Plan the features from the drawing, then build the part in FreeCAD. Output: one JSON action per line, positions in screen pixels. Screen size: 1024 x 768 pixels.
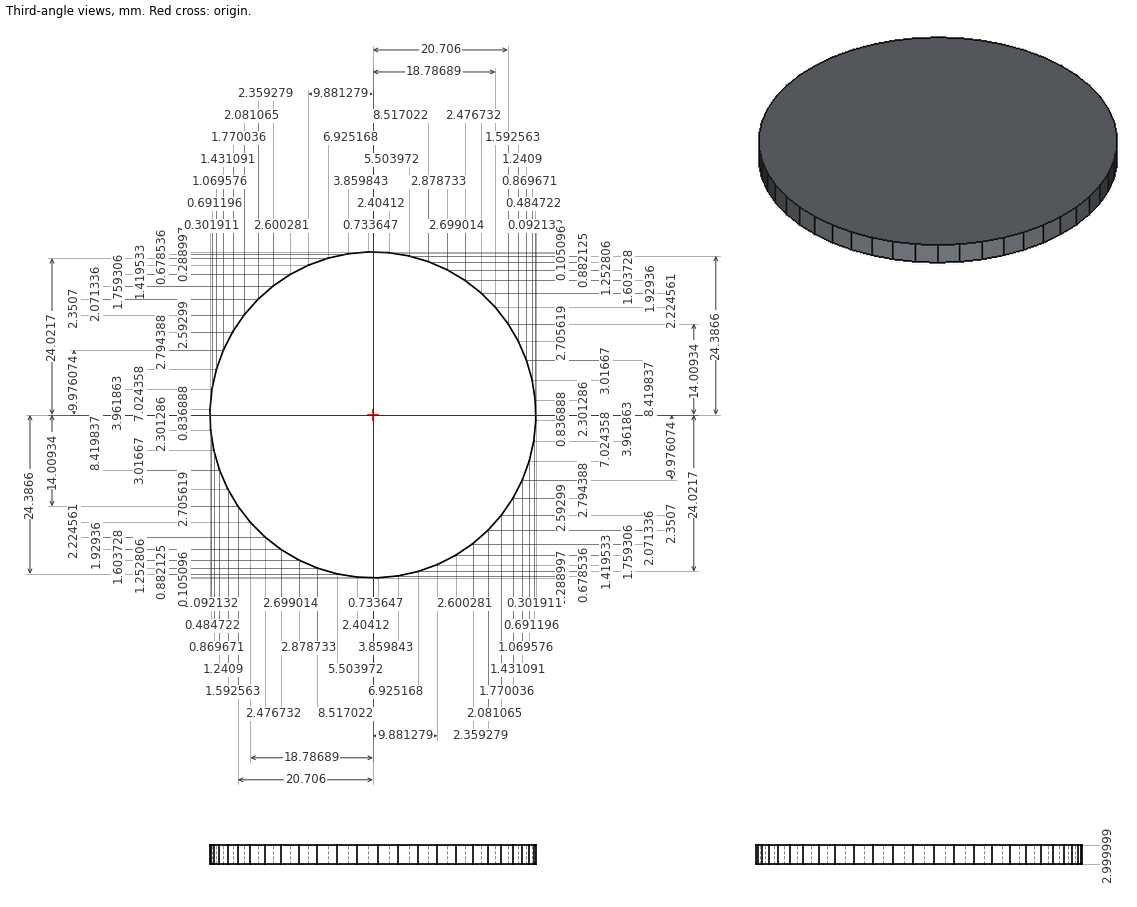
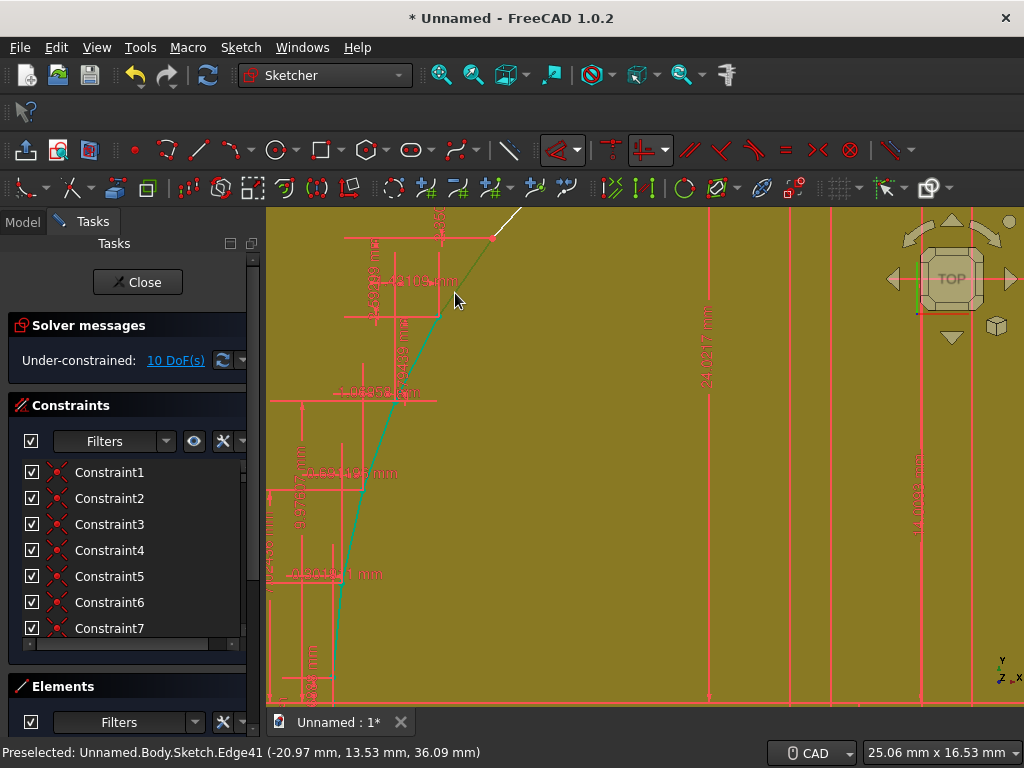
{"action": "key", "text": "l"}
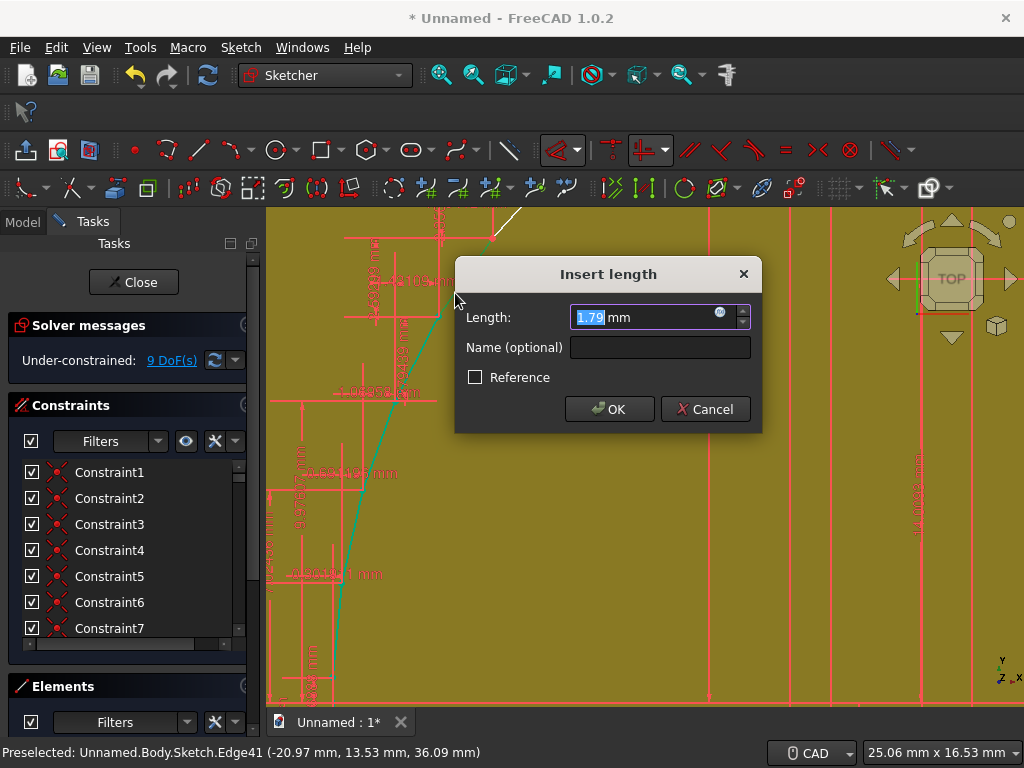
{"action": "type", "text": "1.770036"}
{"action": "key", "text": "Return"}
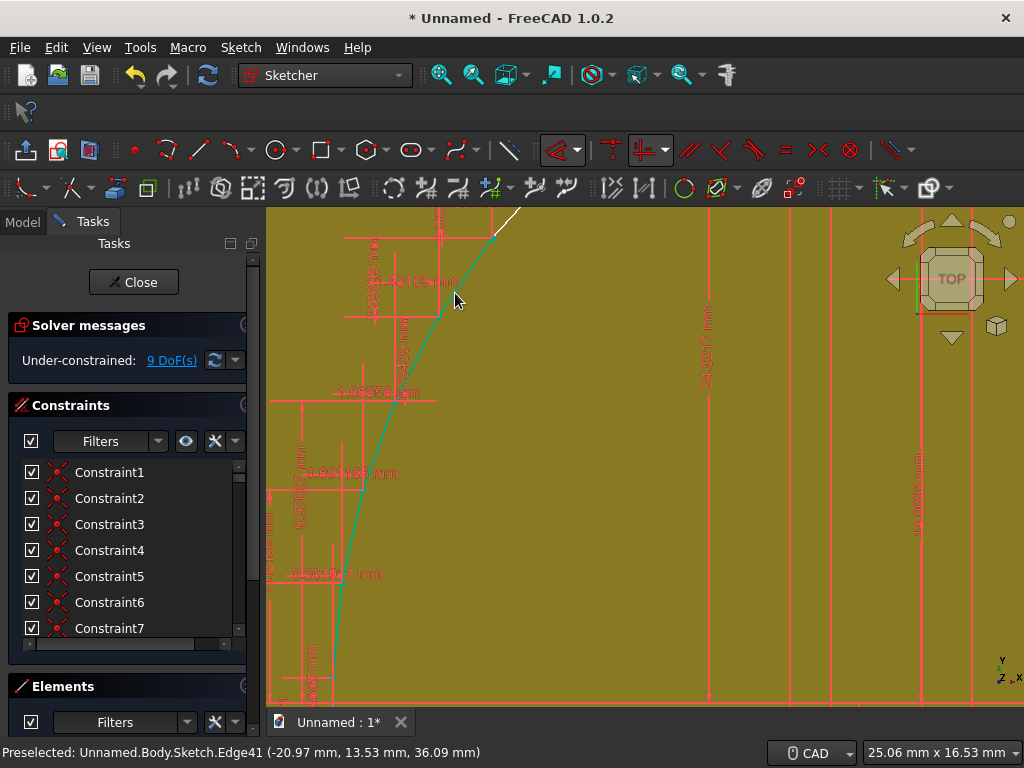
{"action": "scroll", "coordinate": [447, 395], "scroll_direction": "down", "scroll_amount": 8}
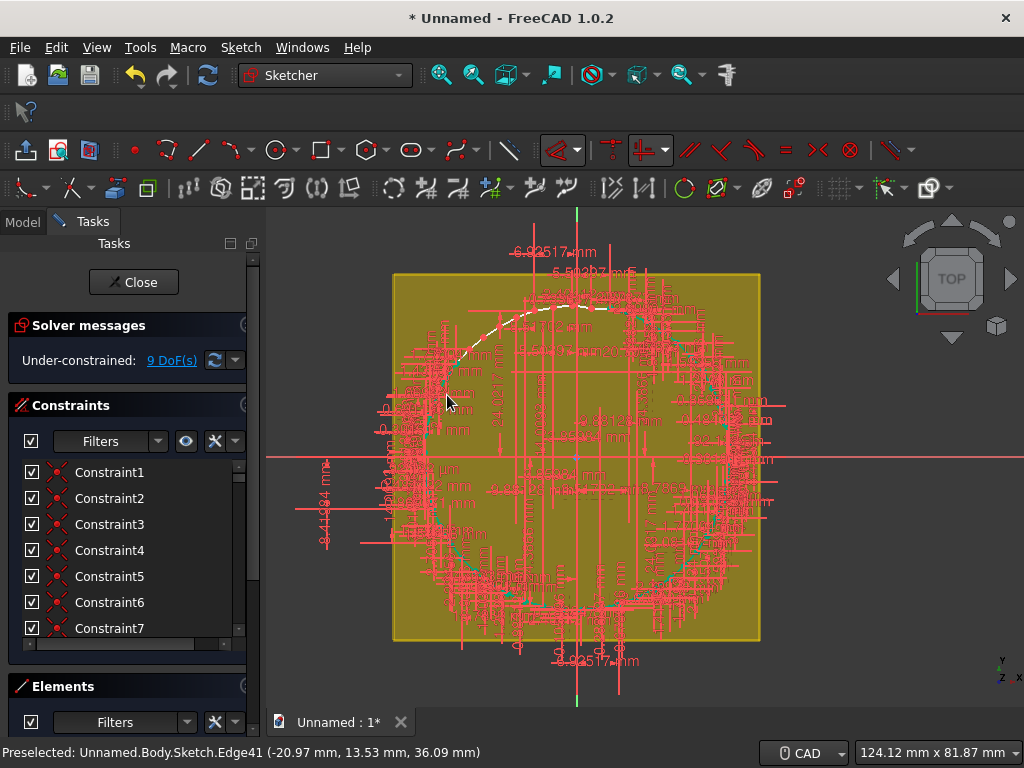
{"action": "scroll", "coordinate": [460, 359], "scroll_direction": "up", "scroll_amount": 6}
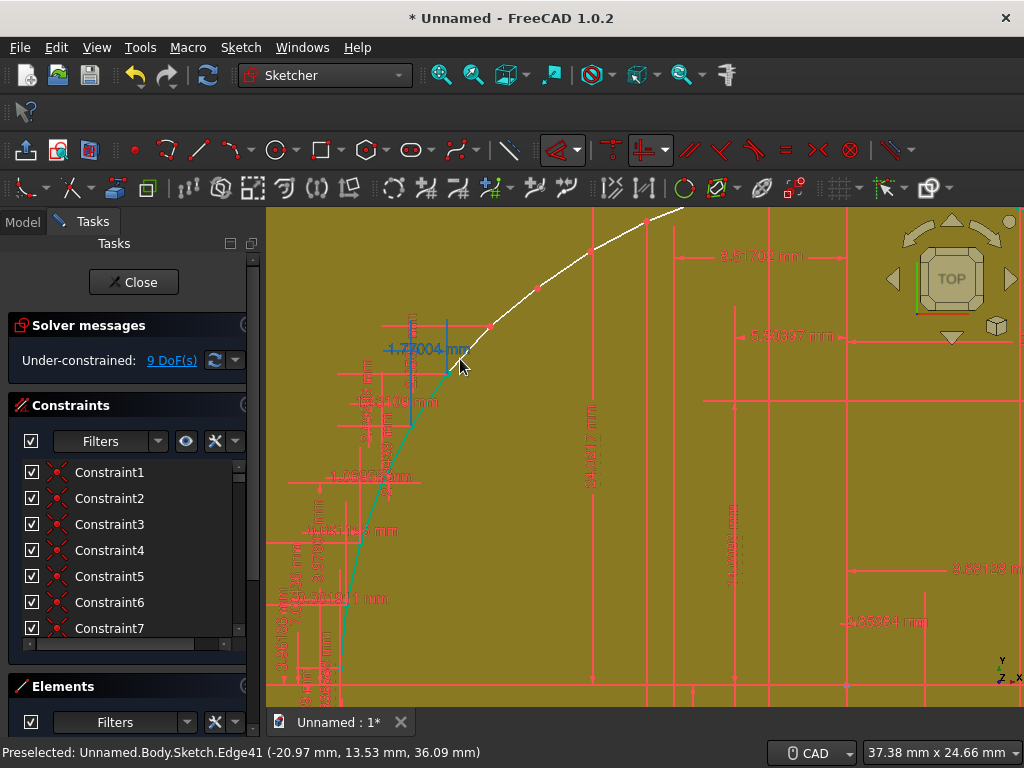
{"action": "left_click", "coordinate": [460, 359]}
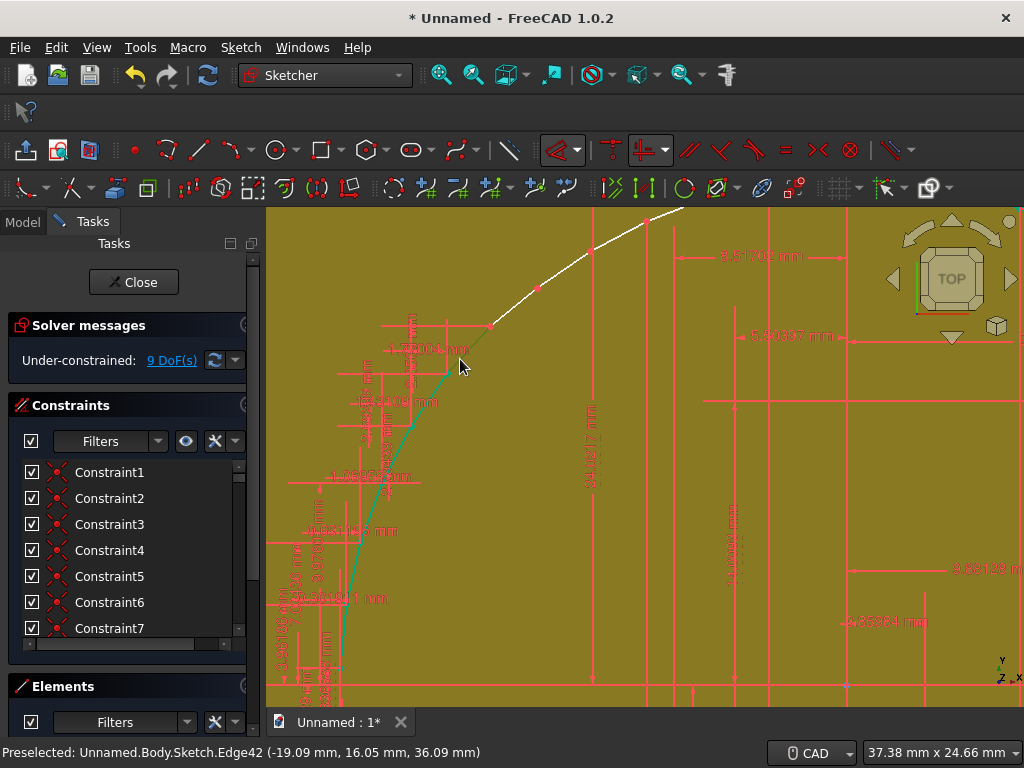
{"action": "left_click", "coordinate": [580, 150]}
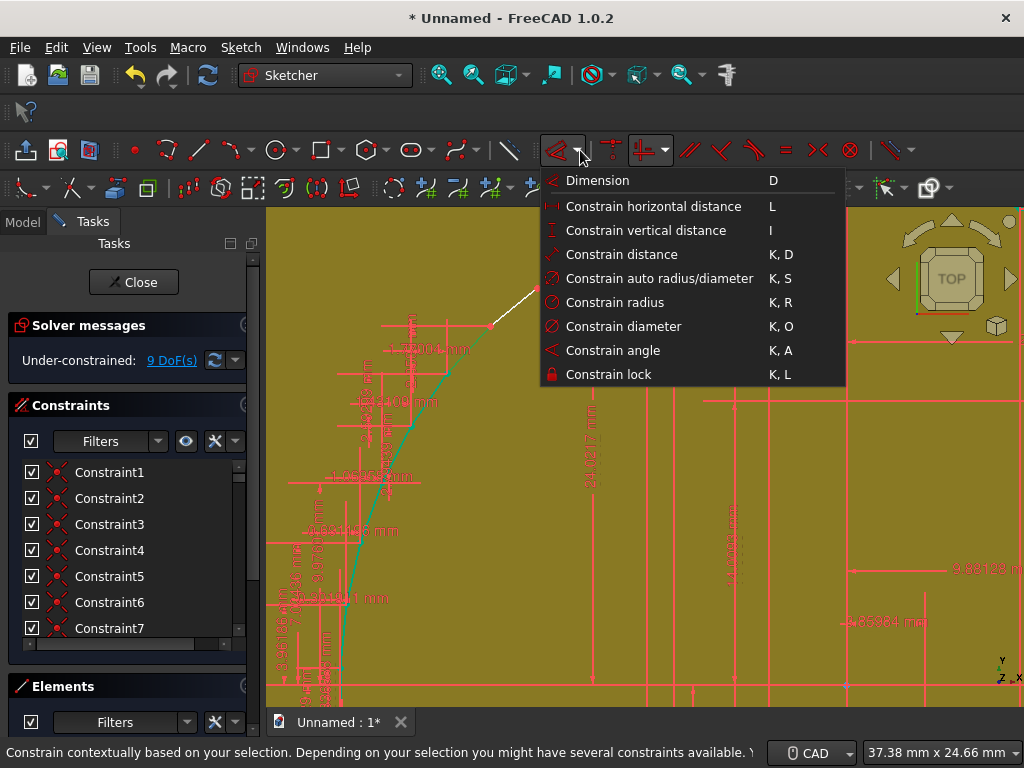
{"action": "left_click", "coordinate": [693, 206]}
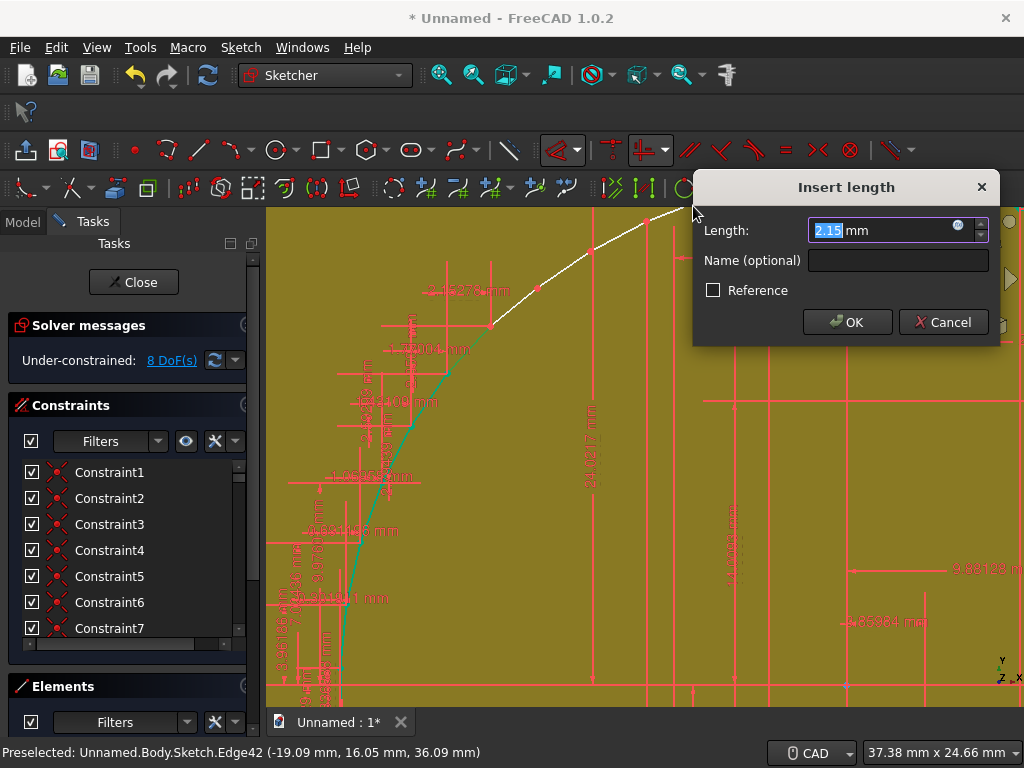
{"action": "type", "text": "2.081065"}
{"action": "key", "text": "Return"}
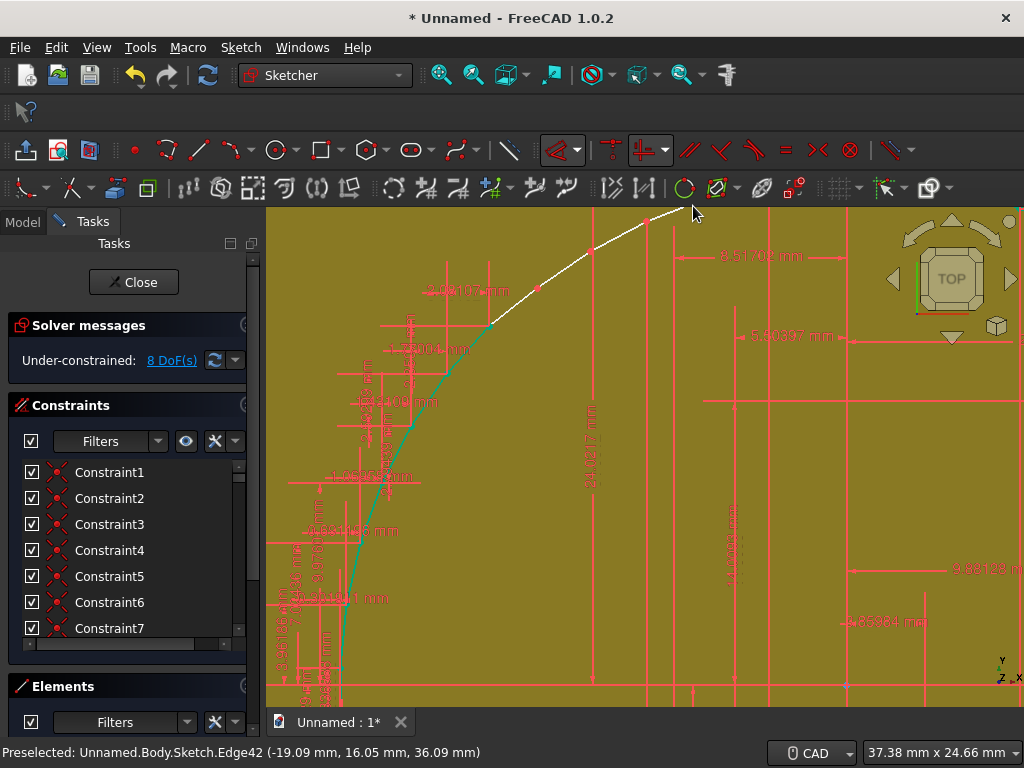
{"action": "left_click", "coordinate": [504, 315]}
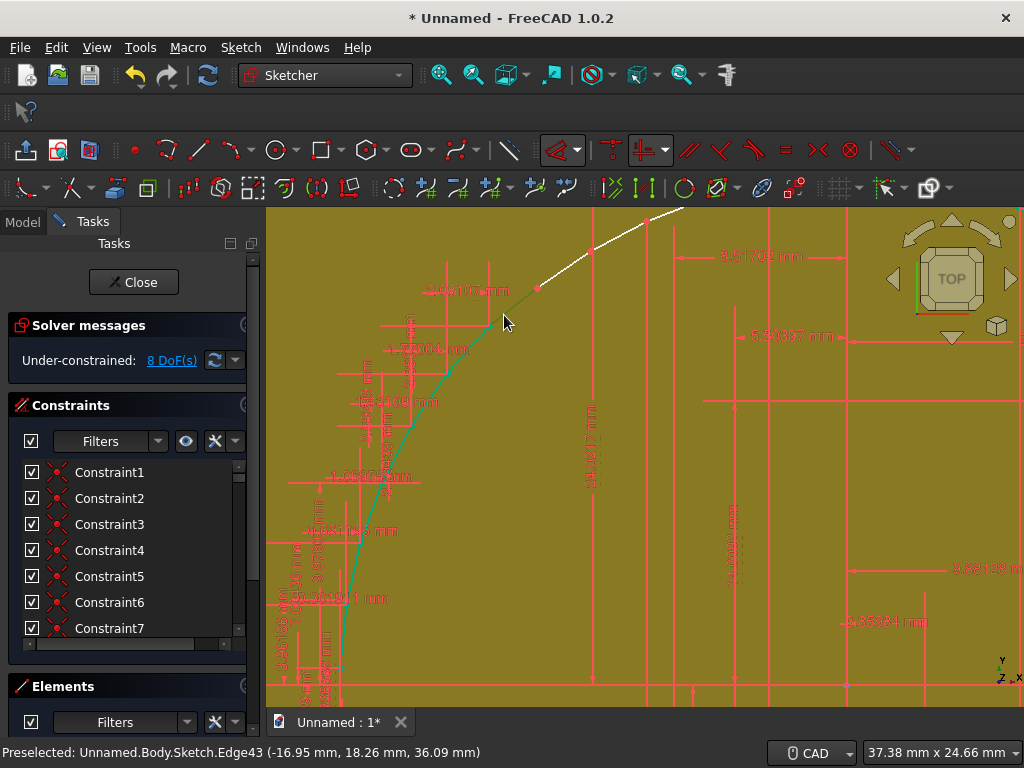
{"action": "left_click", "coordinate": [580, 150]}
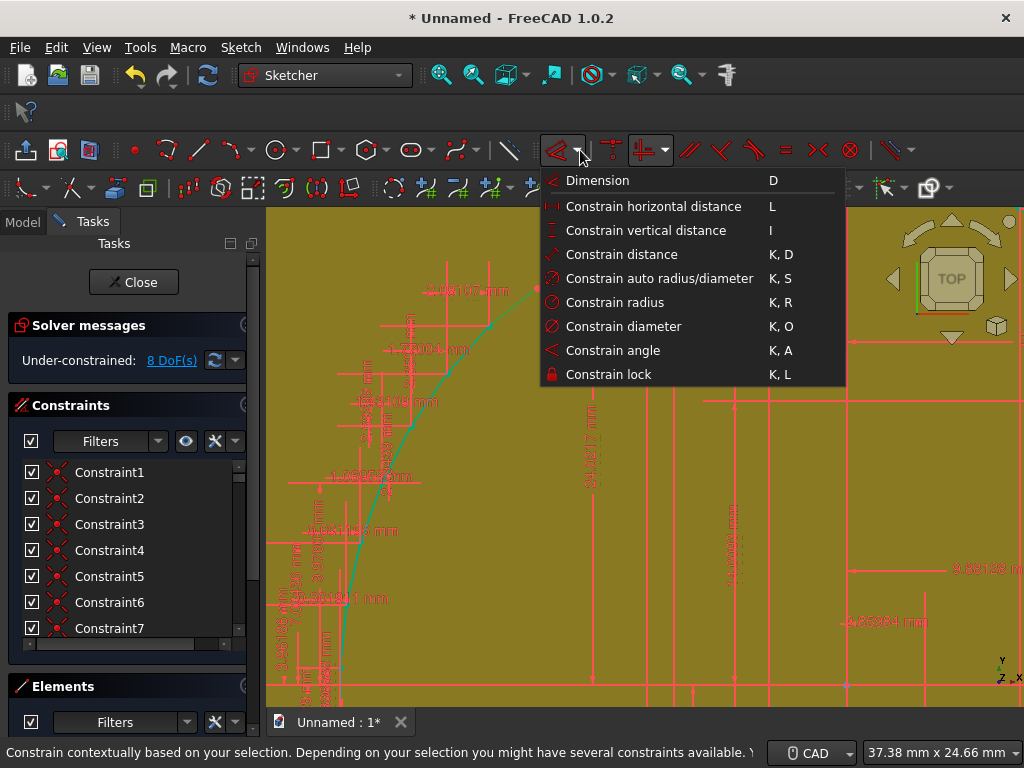
{"action": "left_click", "coordinate": [693, 206]}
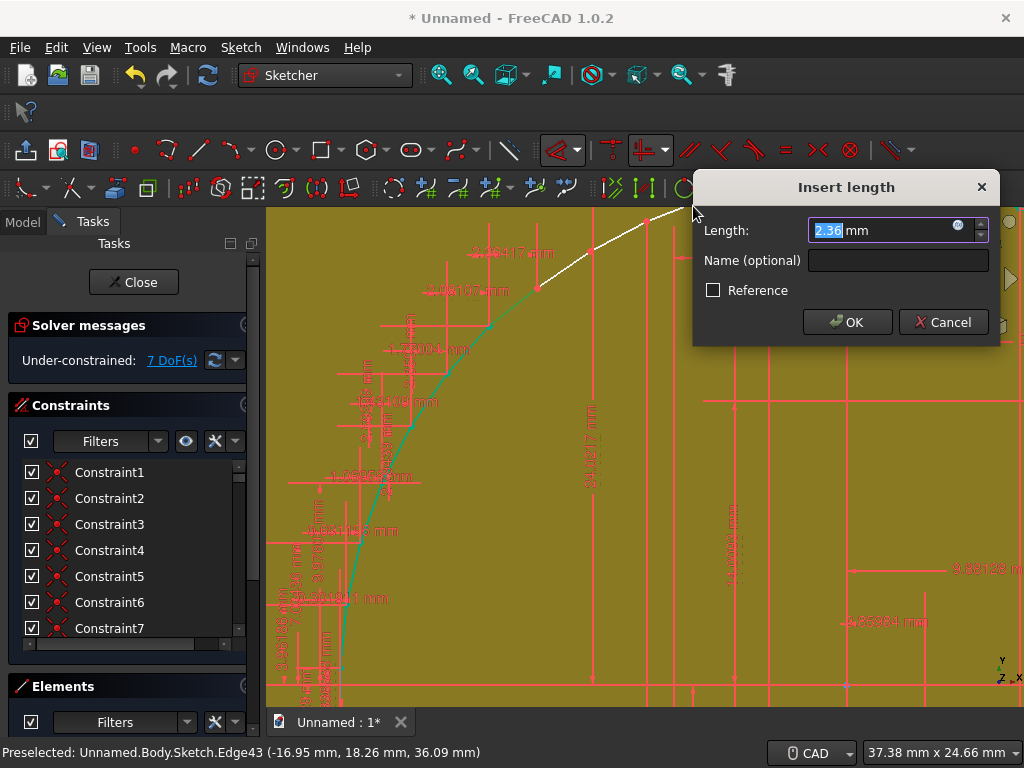
{"action": "type", "text": "2.359279"}
{"action": "key", "text": "Return"}